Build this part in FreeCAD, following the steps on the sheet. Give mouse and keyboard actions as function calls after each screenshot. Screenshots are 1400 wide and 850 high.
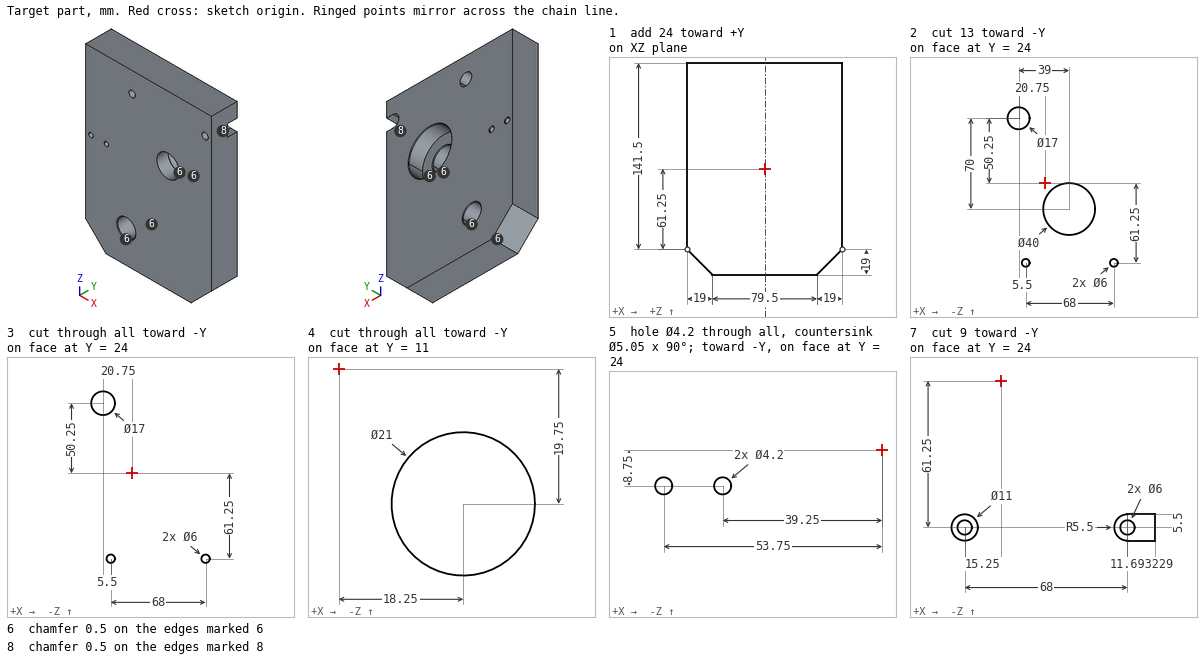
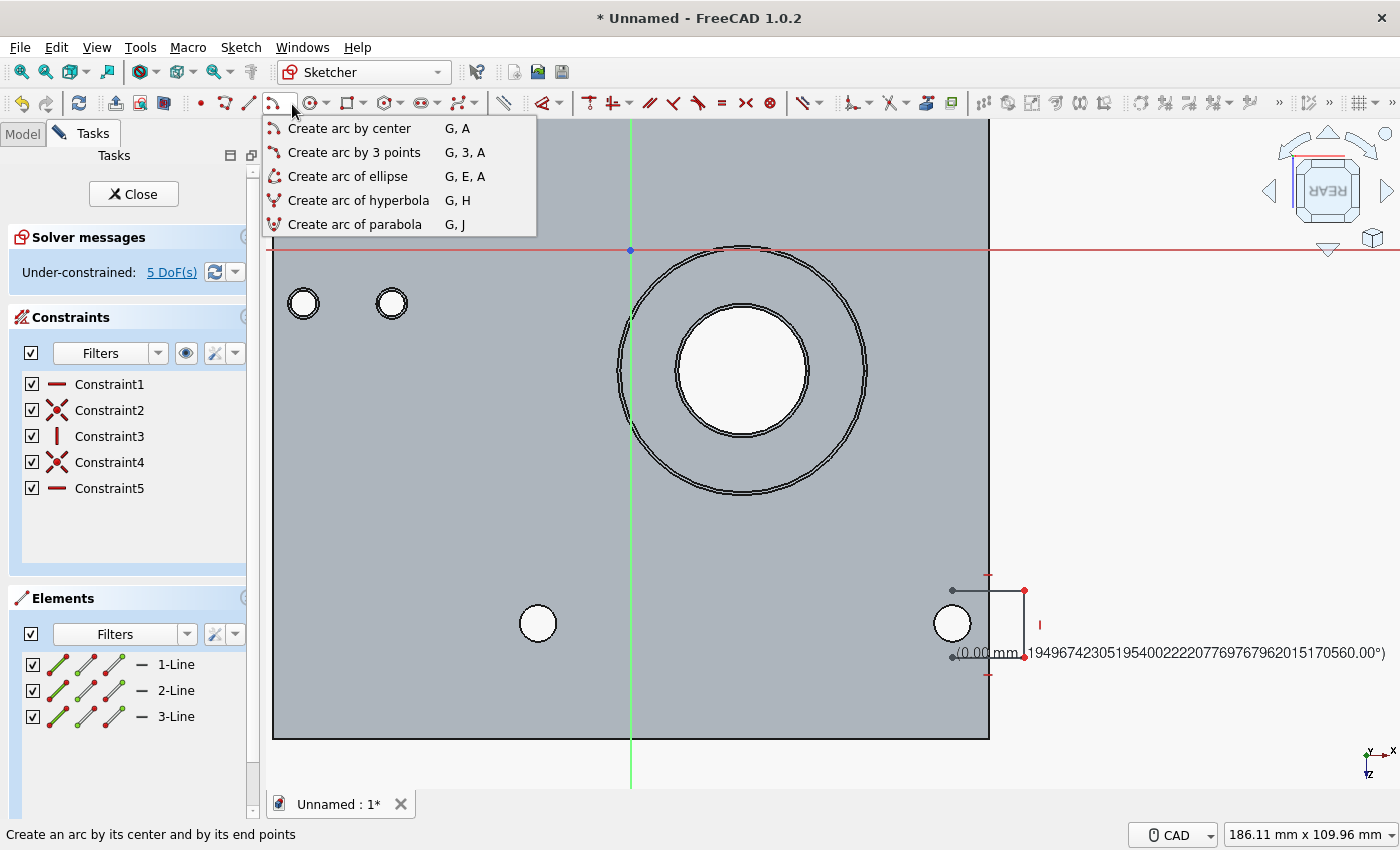
click(400, 152)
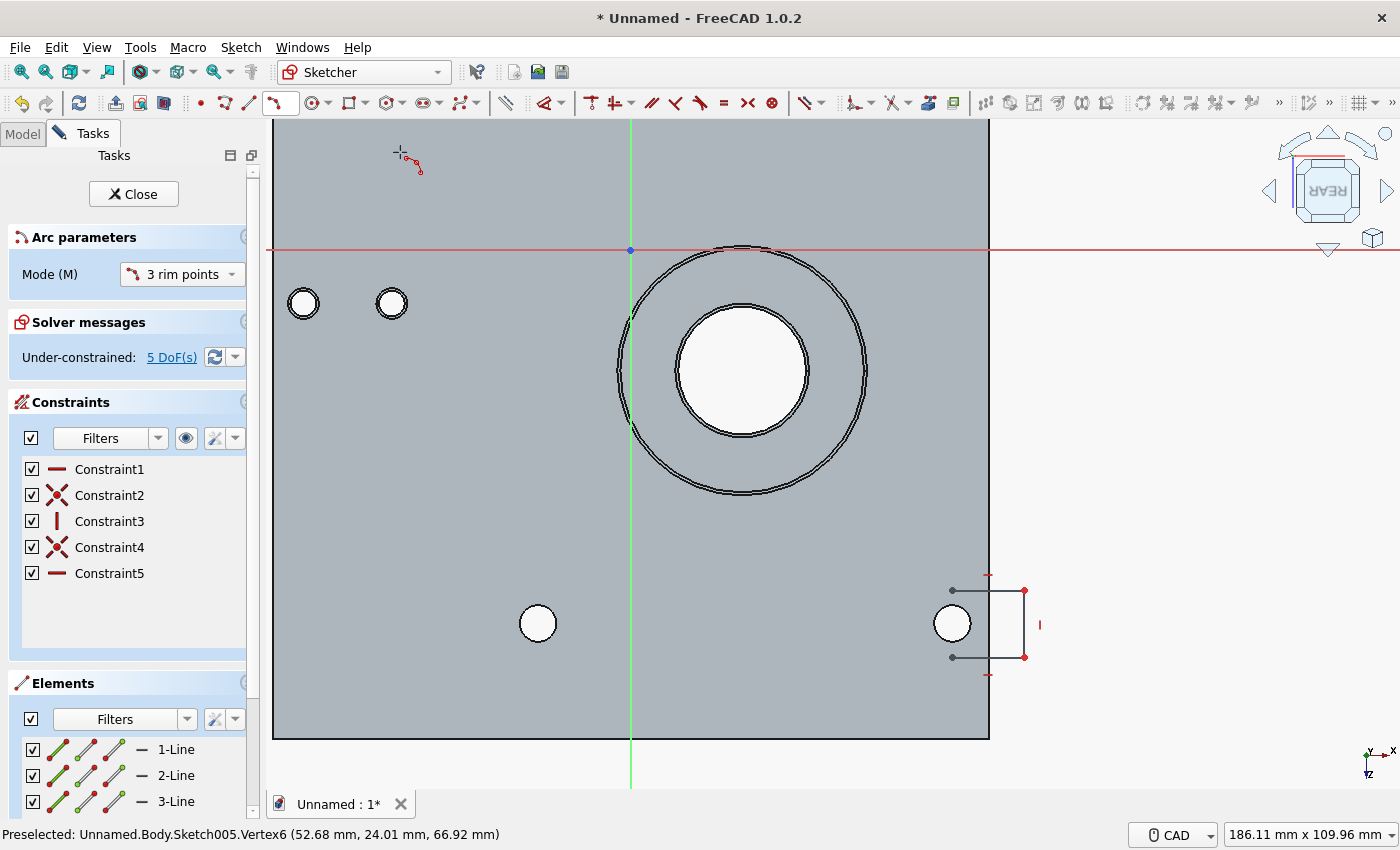
click(952, 658)
click(952, 591)
click(919, 623)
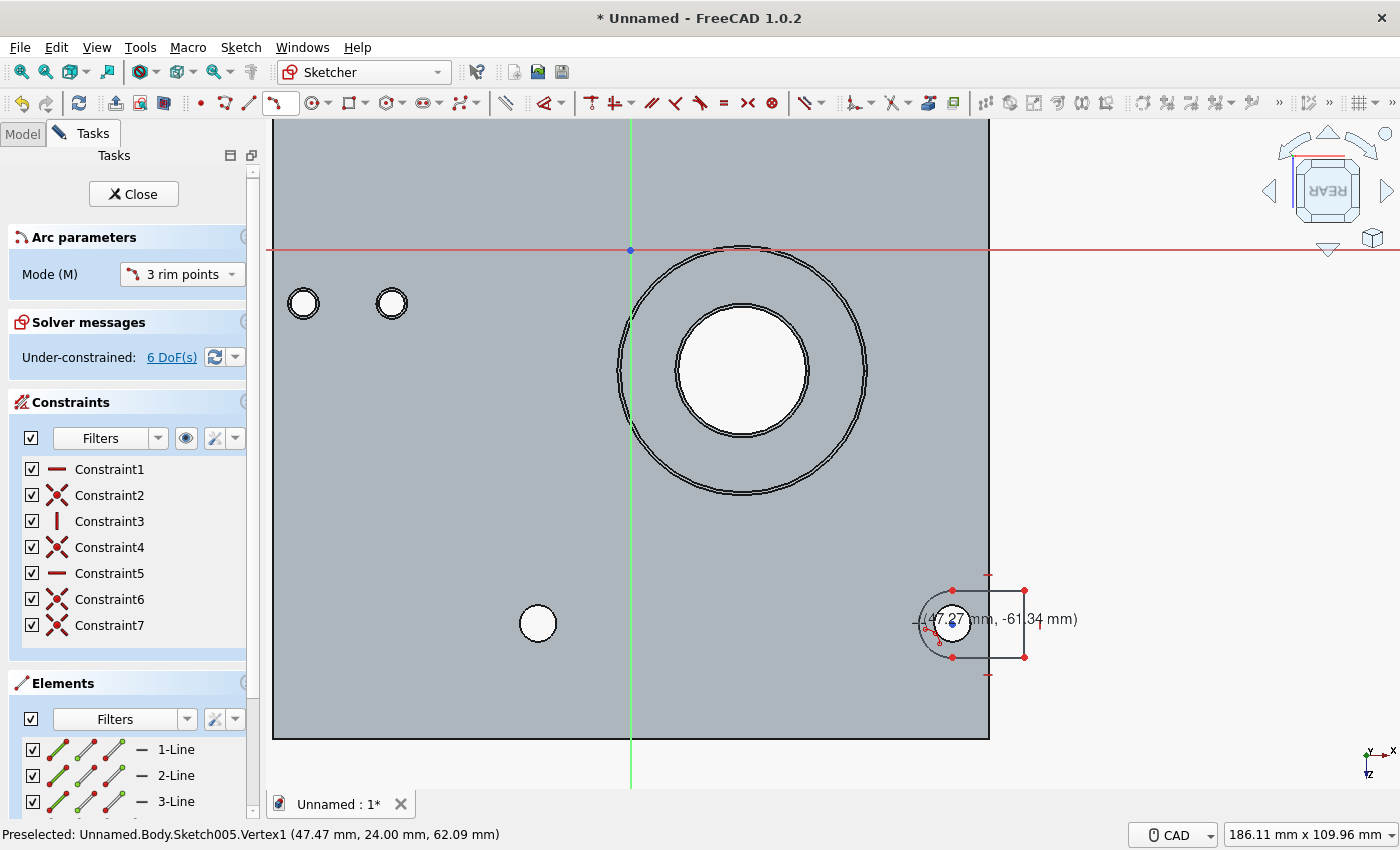
key(g)
key(c)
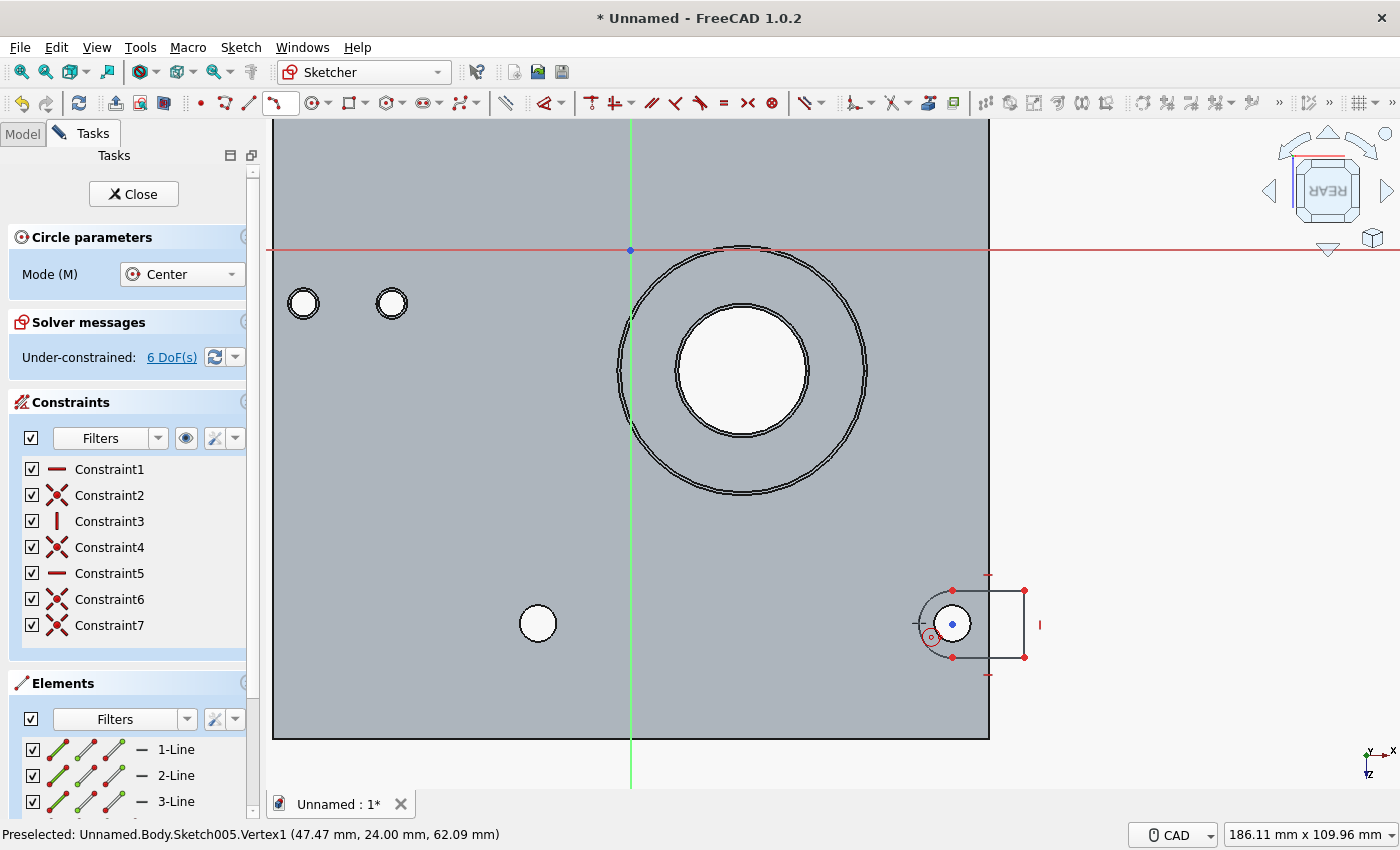
click(538, 623)
move(562, 600)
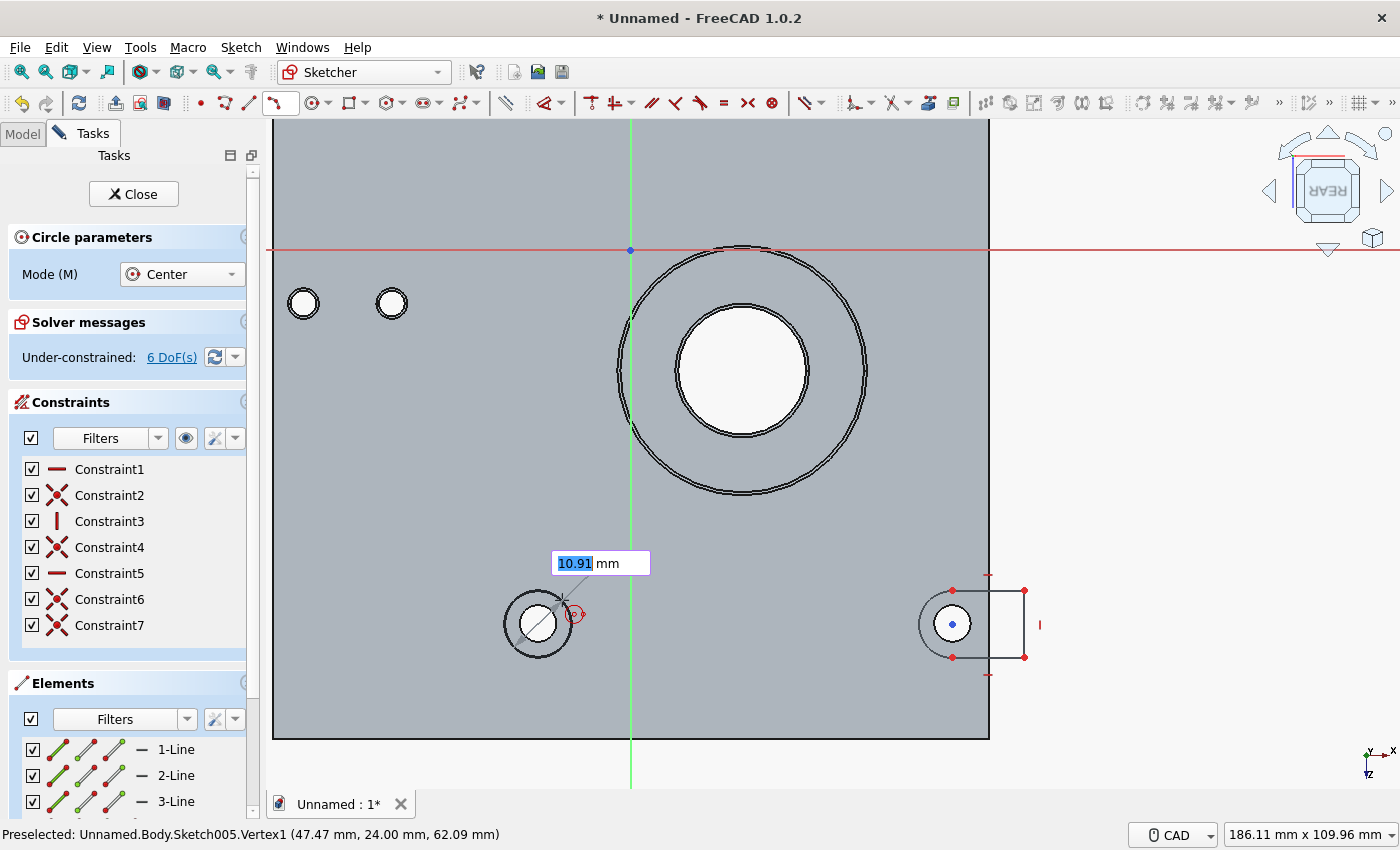
text(11)
key(Return)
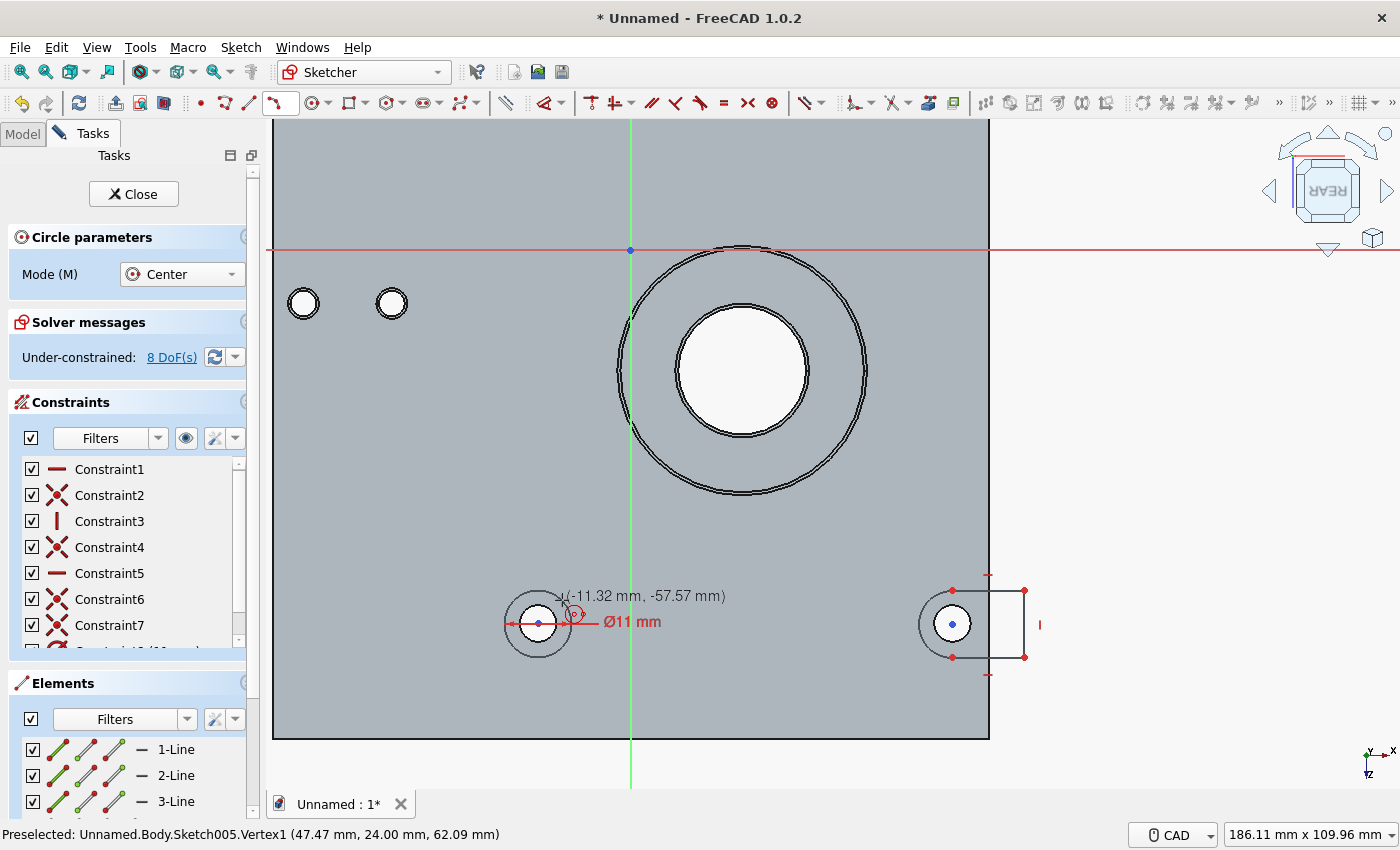
scroll(538, 623, up, 2)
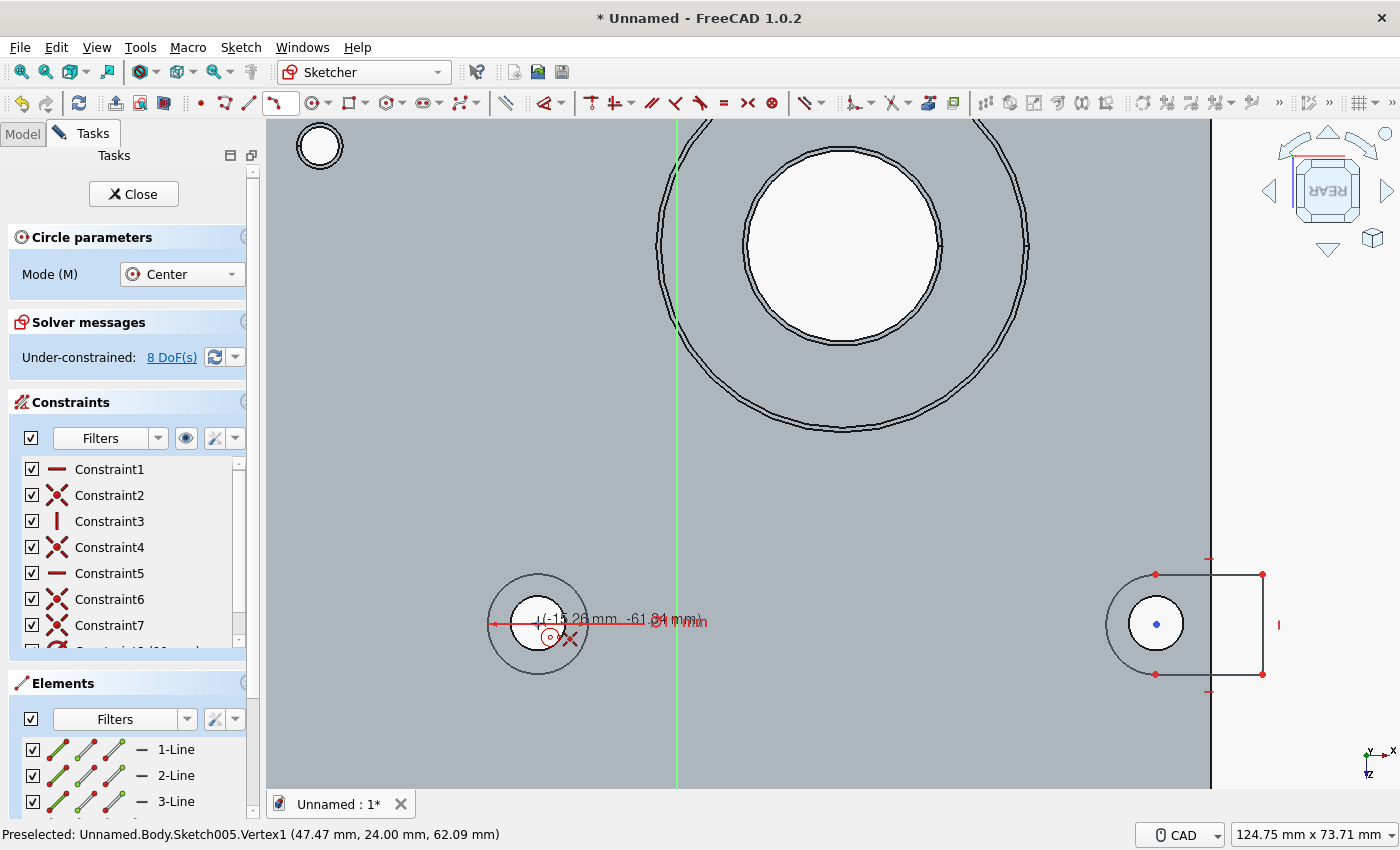
click(538, 624)
move(557, 604)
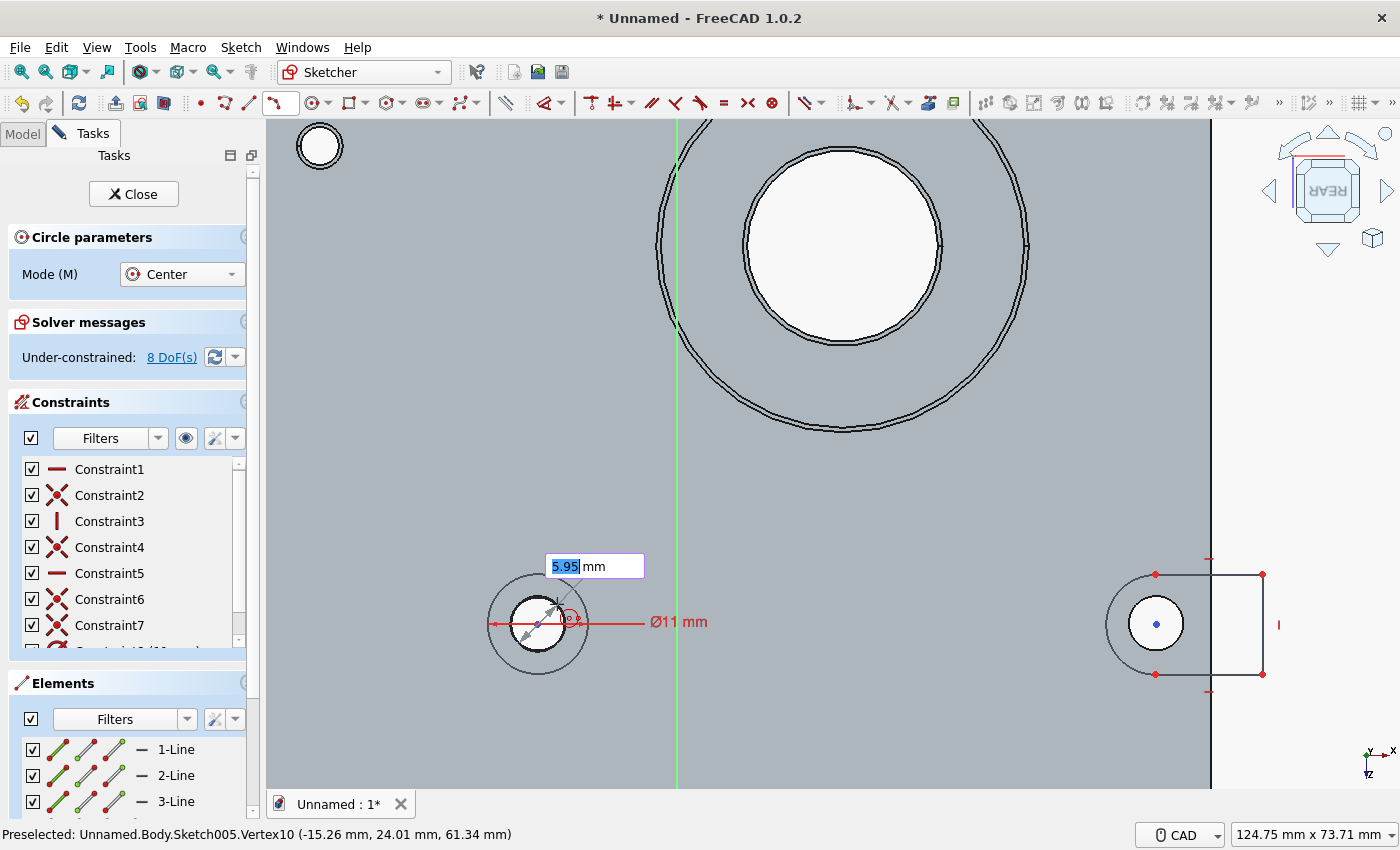
text(6)
key(Return)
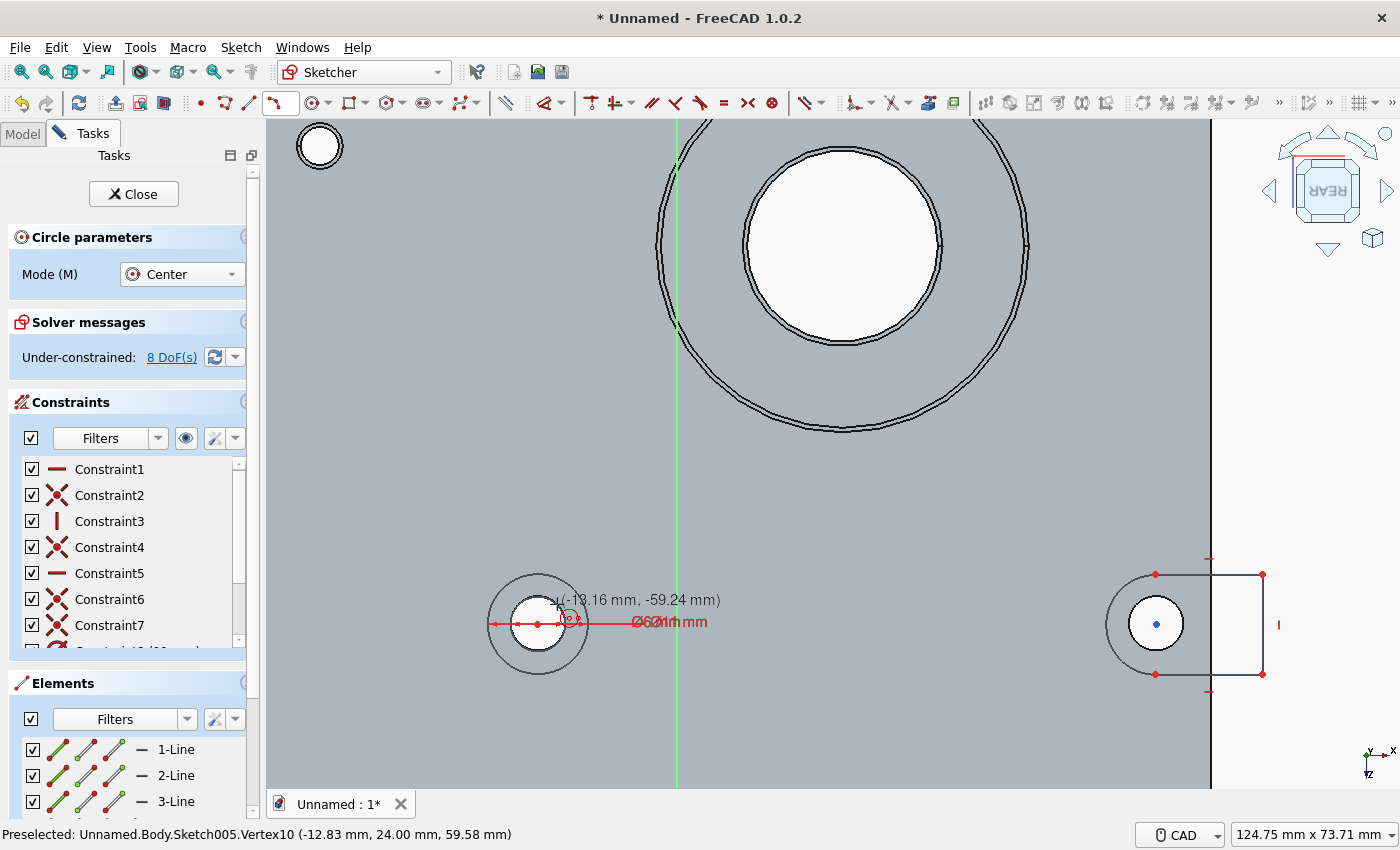
click(1156, 623)
move(1175, 604)